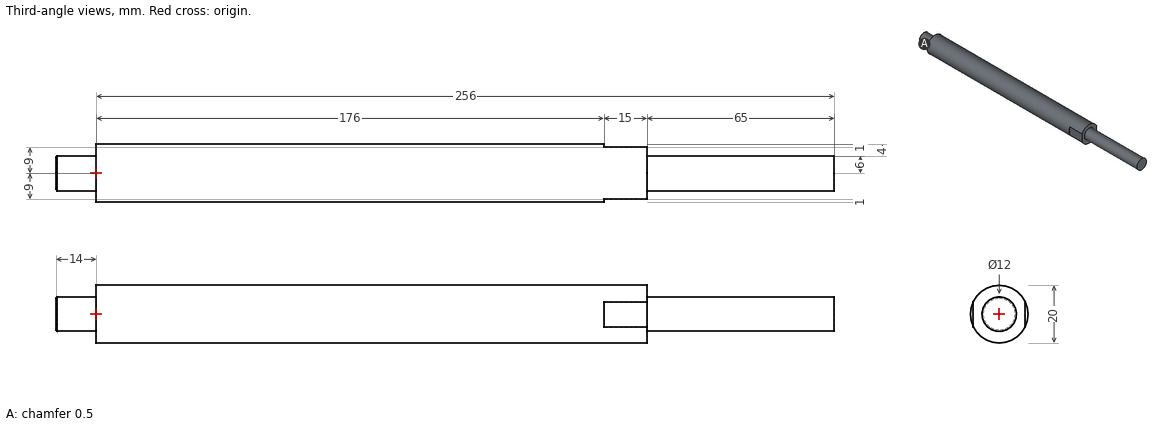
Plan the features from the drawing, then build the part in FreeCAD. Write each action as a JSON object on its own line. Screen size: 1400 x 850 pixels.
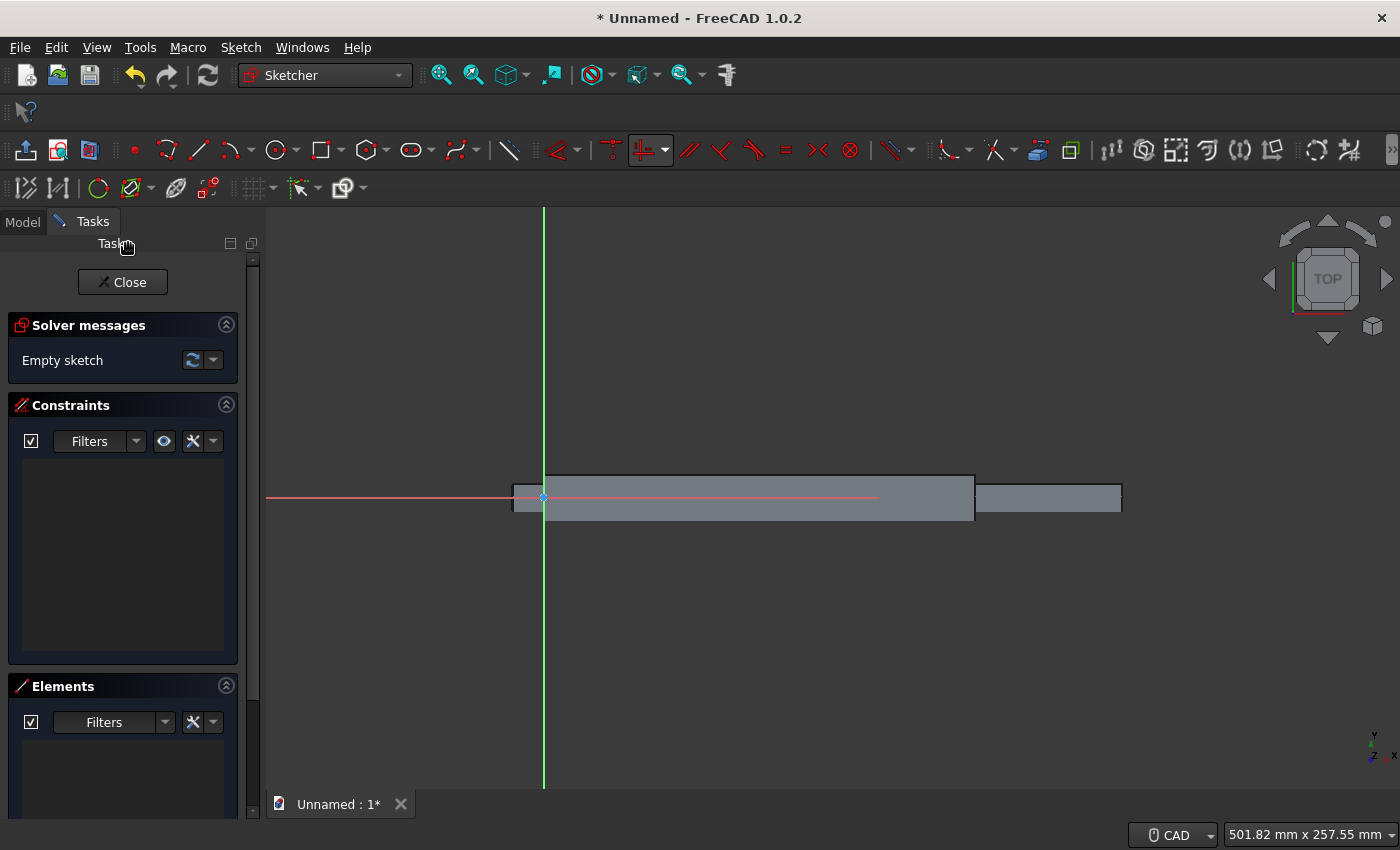
{"action": "scroll", "coordinate": [983, 498], "scroll_direction": "up", "scroll_amount": 11}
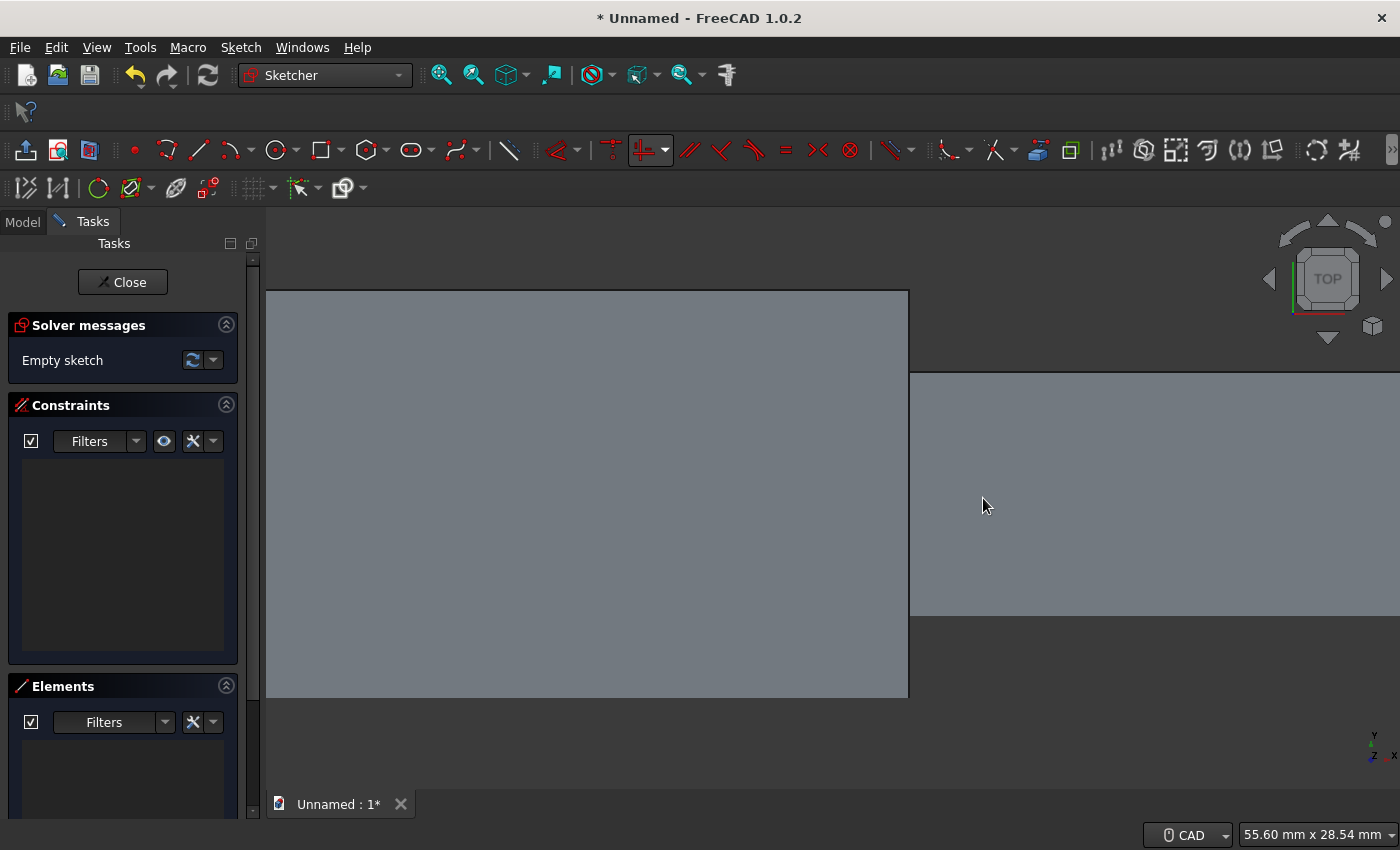
{"action": "key", "text": "g r"}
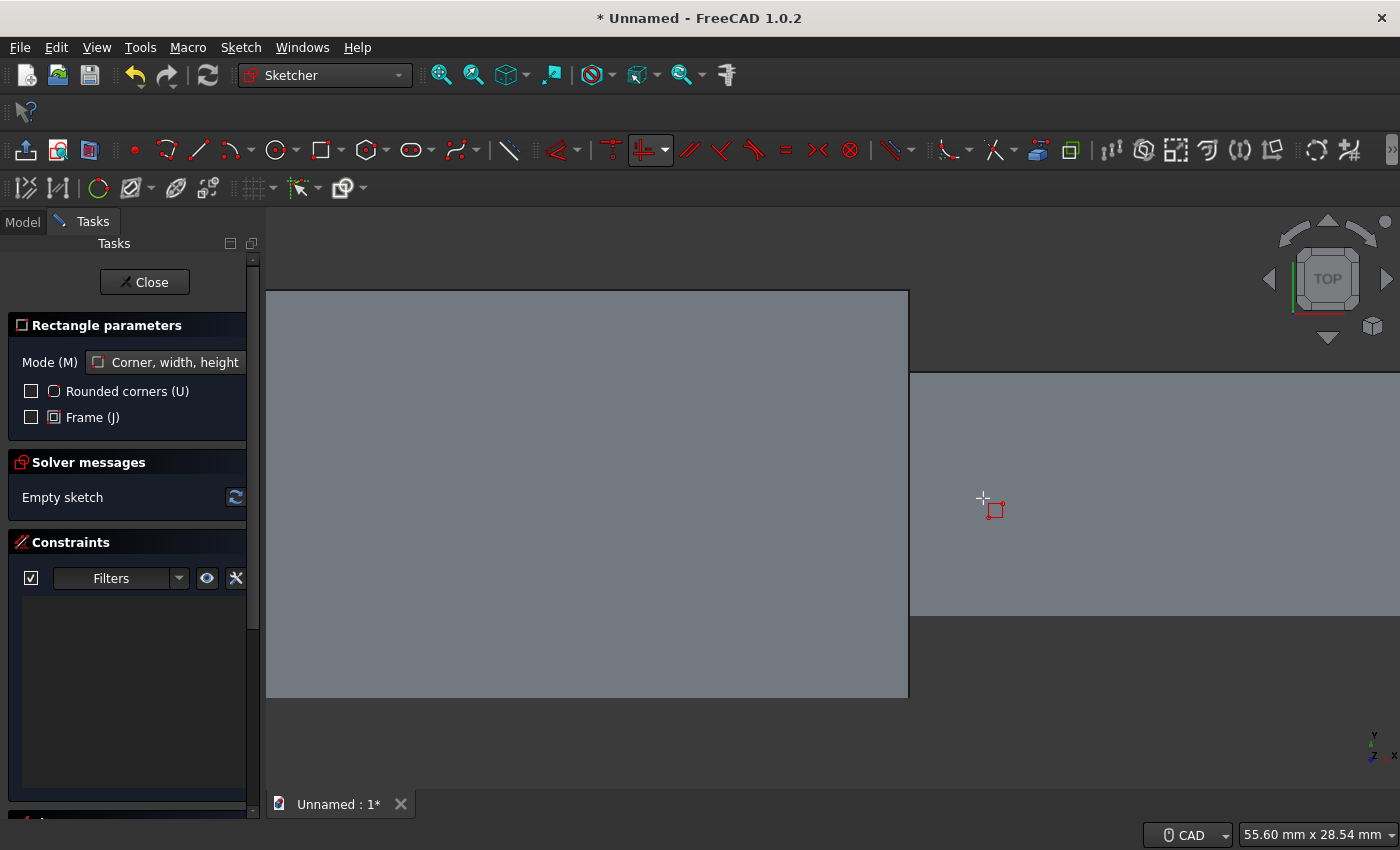
{"action": "left_click", "coordinate": [603, 290]}
{"action": "mouse_move", "coordinate": [909, 310]}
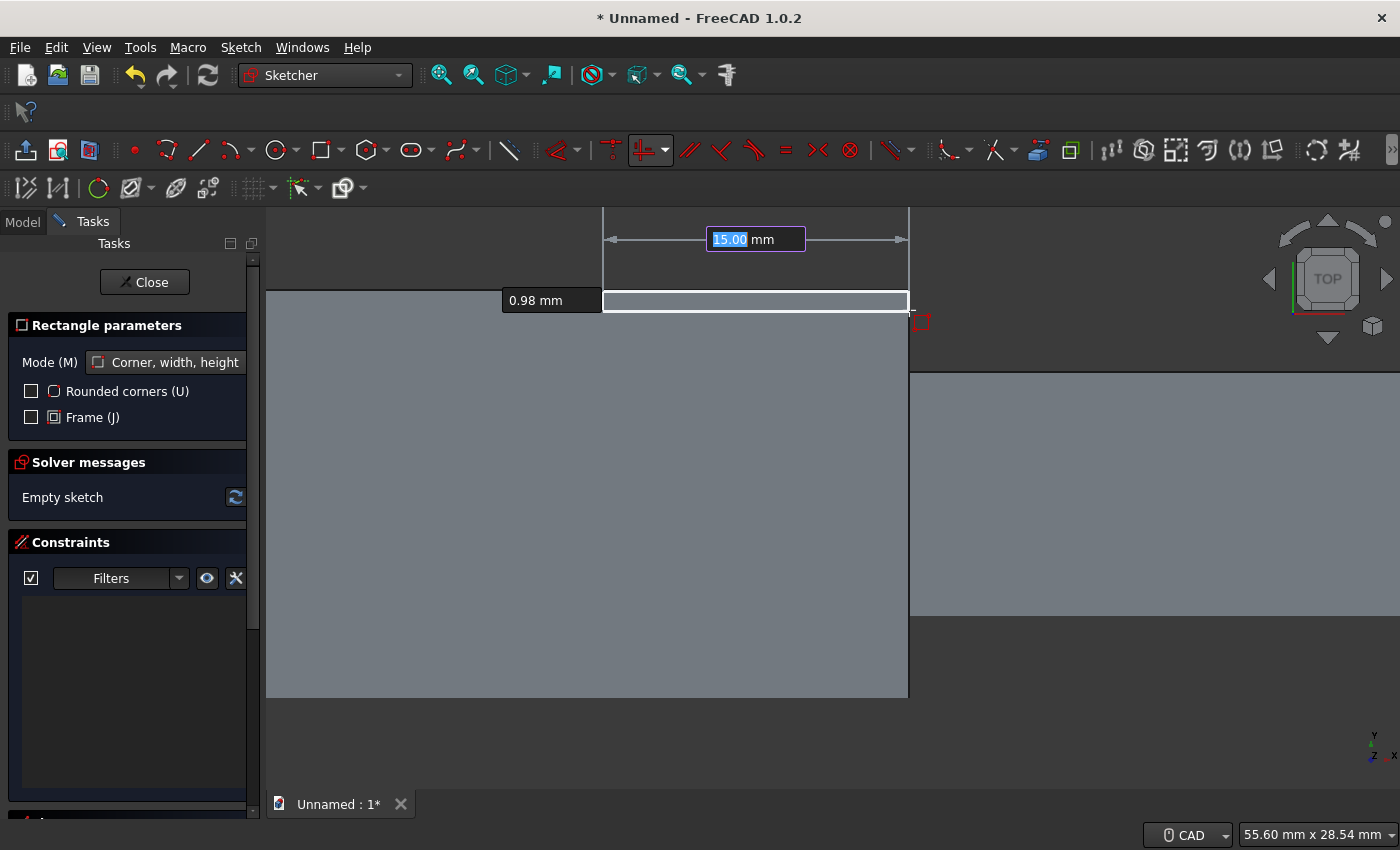
{"action": "type", "text": "15"}
{"action": "key", "text": "Tab"}
{"action": "type", "text": "1"}
{"action": "key", "text": "Return"}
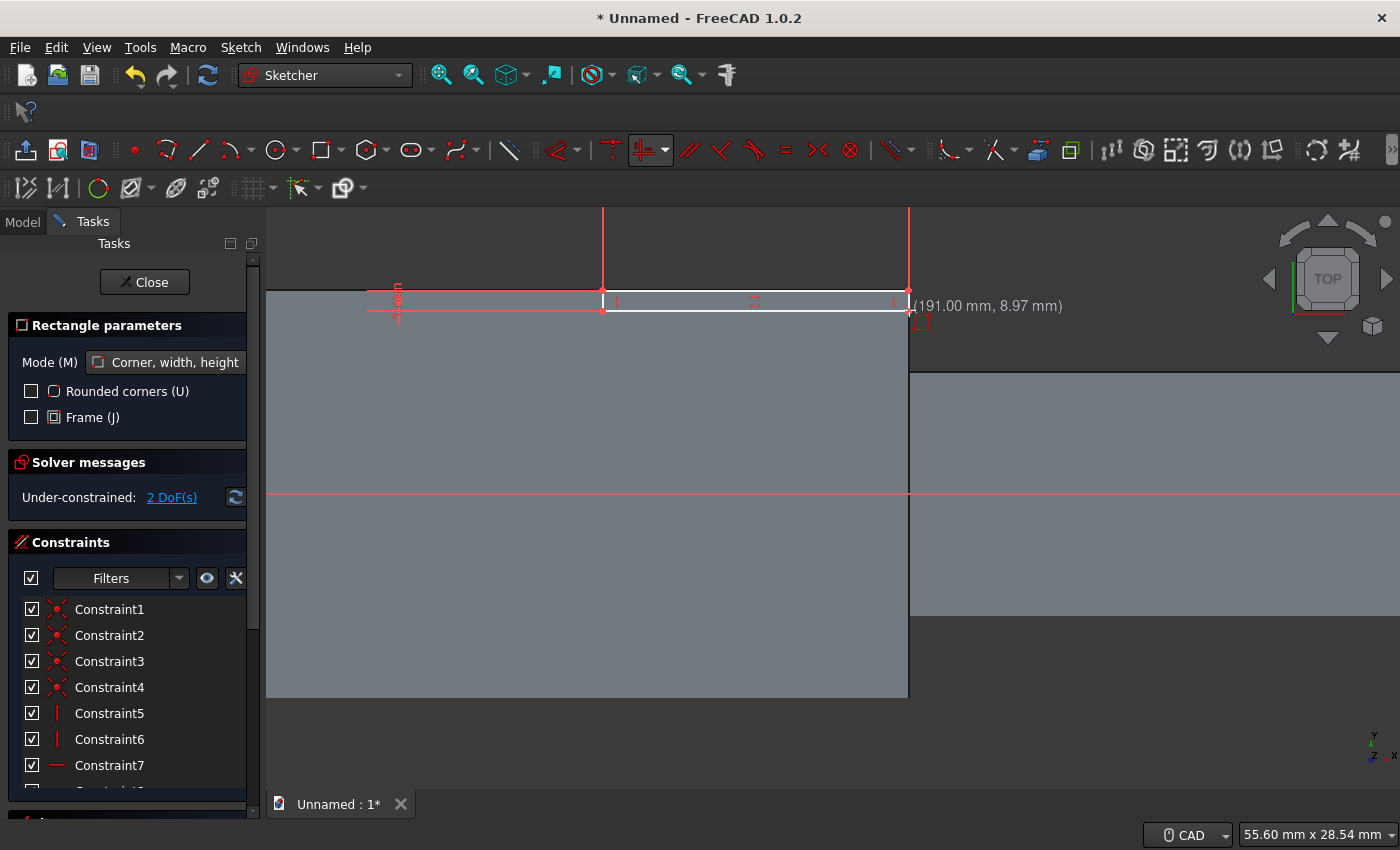
{"action": "left_click", "coordinate": [603, 678]}
{"action": "mouse_move", "coordinate": [909, 698]}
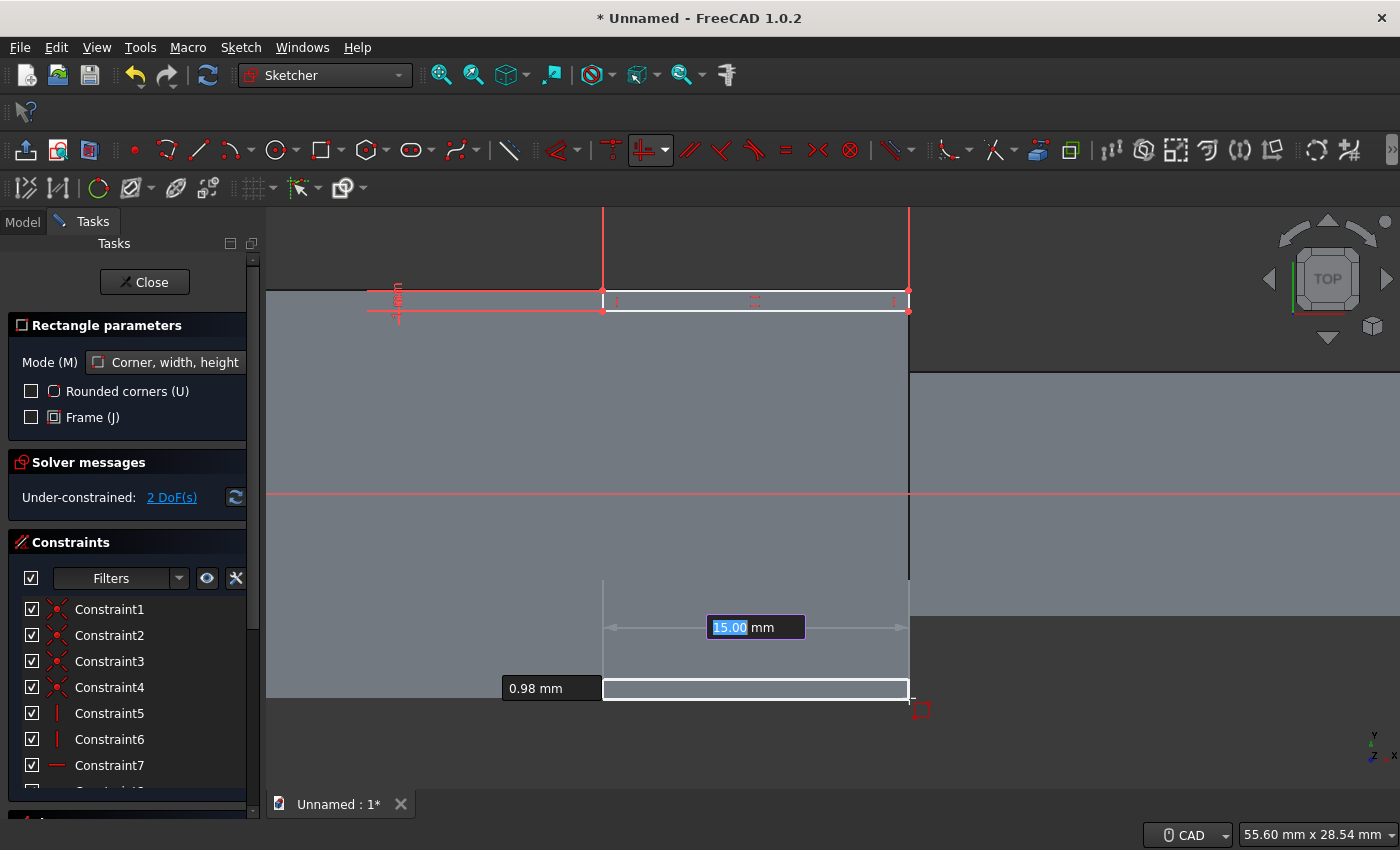
{"action": "type", "text": "15"}
{"action": "key", "text": "Tab"}
{"action": "type", "text": "1"}
{"action": "key", "text": "Return"}
{"action": "key", "text": "Escape"}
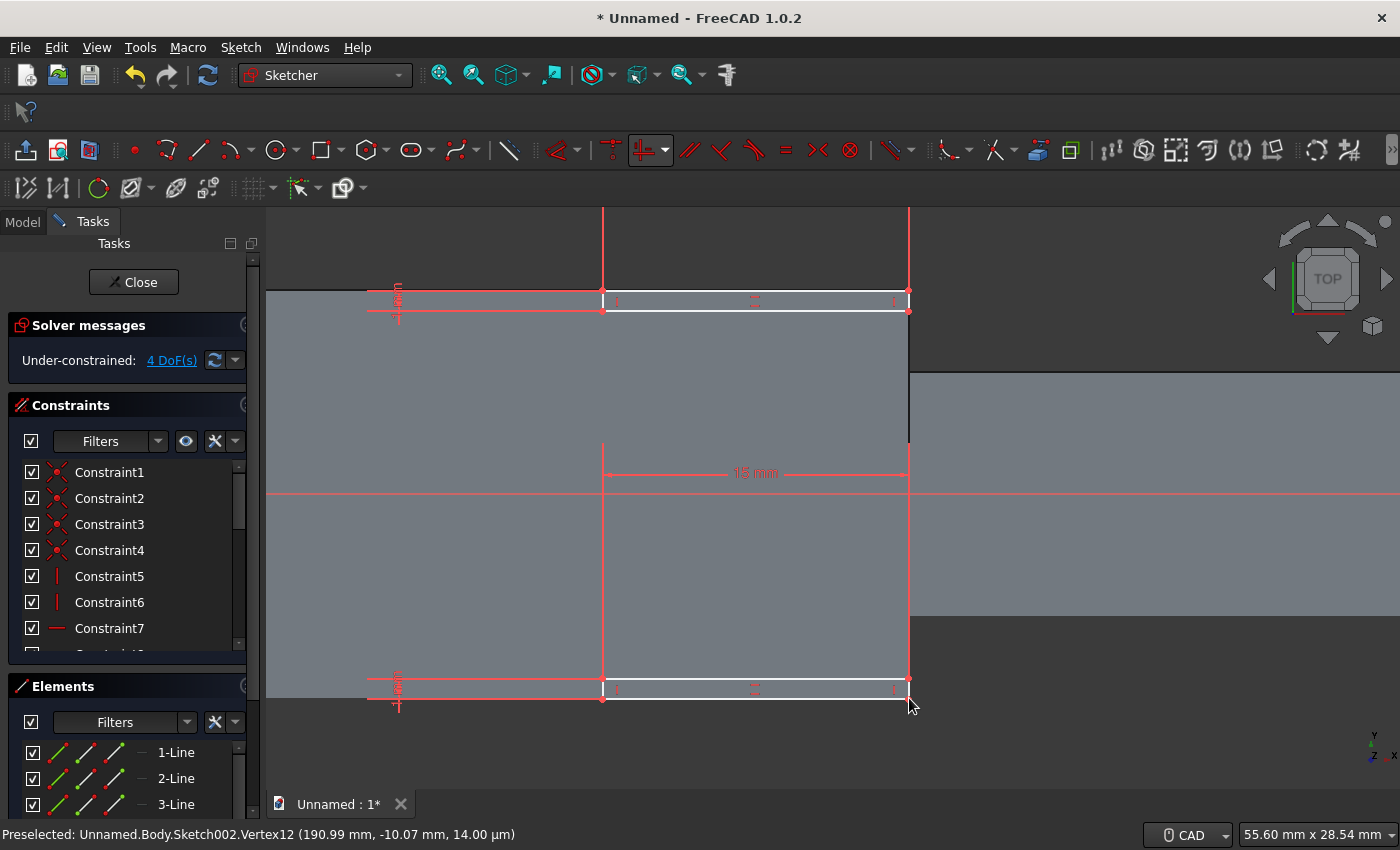
{"action": "key", "text": "d"}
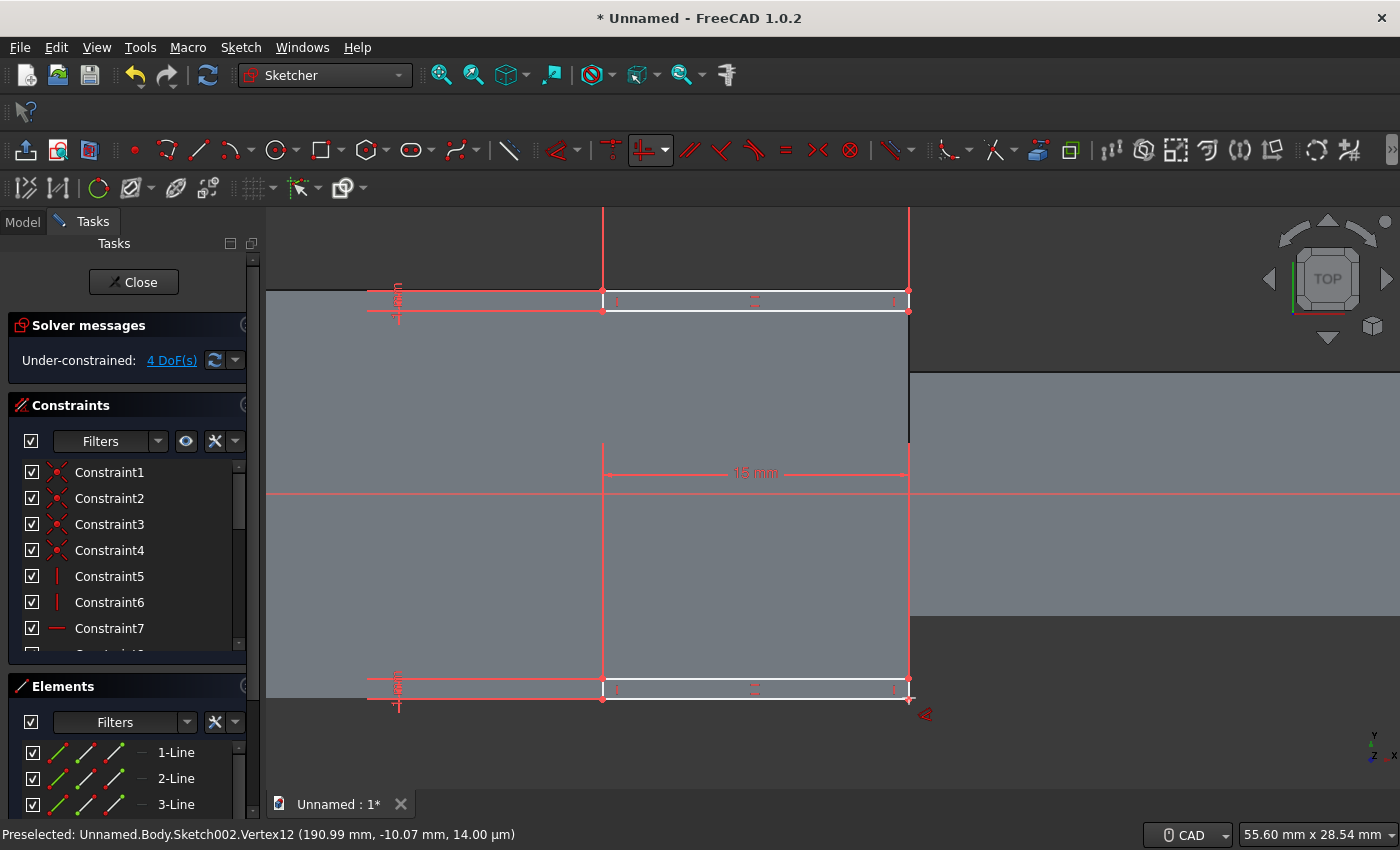
{"action": "left_click", "coordinate": [603, 311]}
{"action": "left_click", "coordinate": [637, 403]}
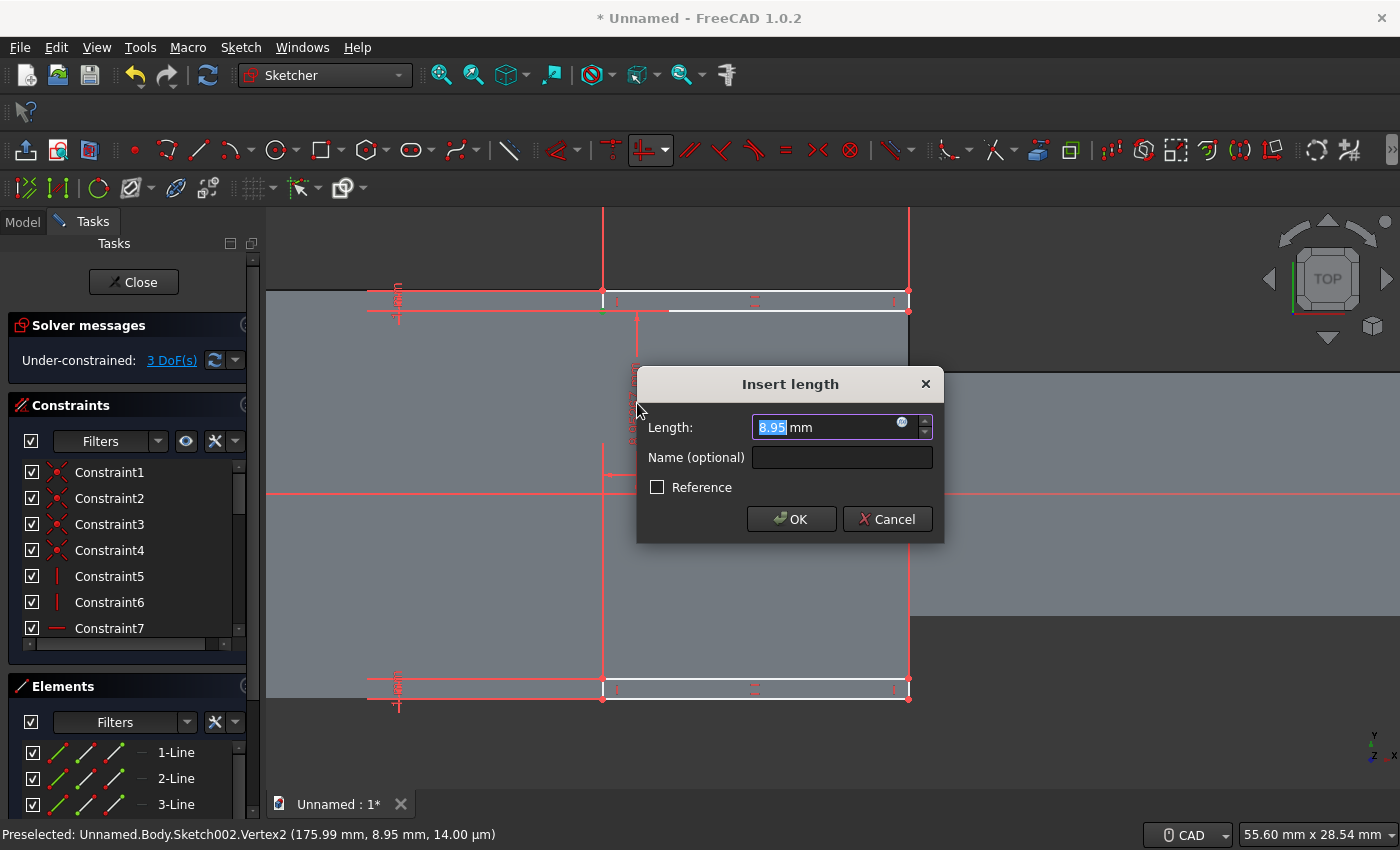
{"action": "type", "text": "9"}
{"action": "key", "text": "Return"}